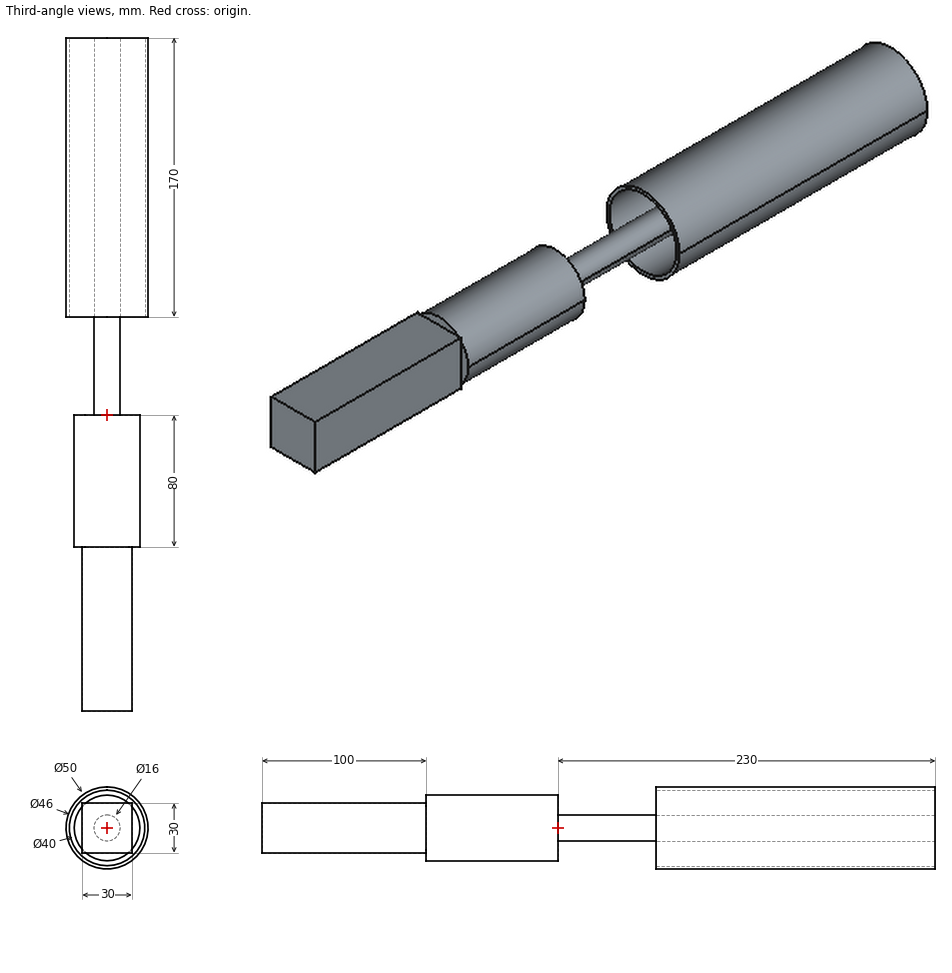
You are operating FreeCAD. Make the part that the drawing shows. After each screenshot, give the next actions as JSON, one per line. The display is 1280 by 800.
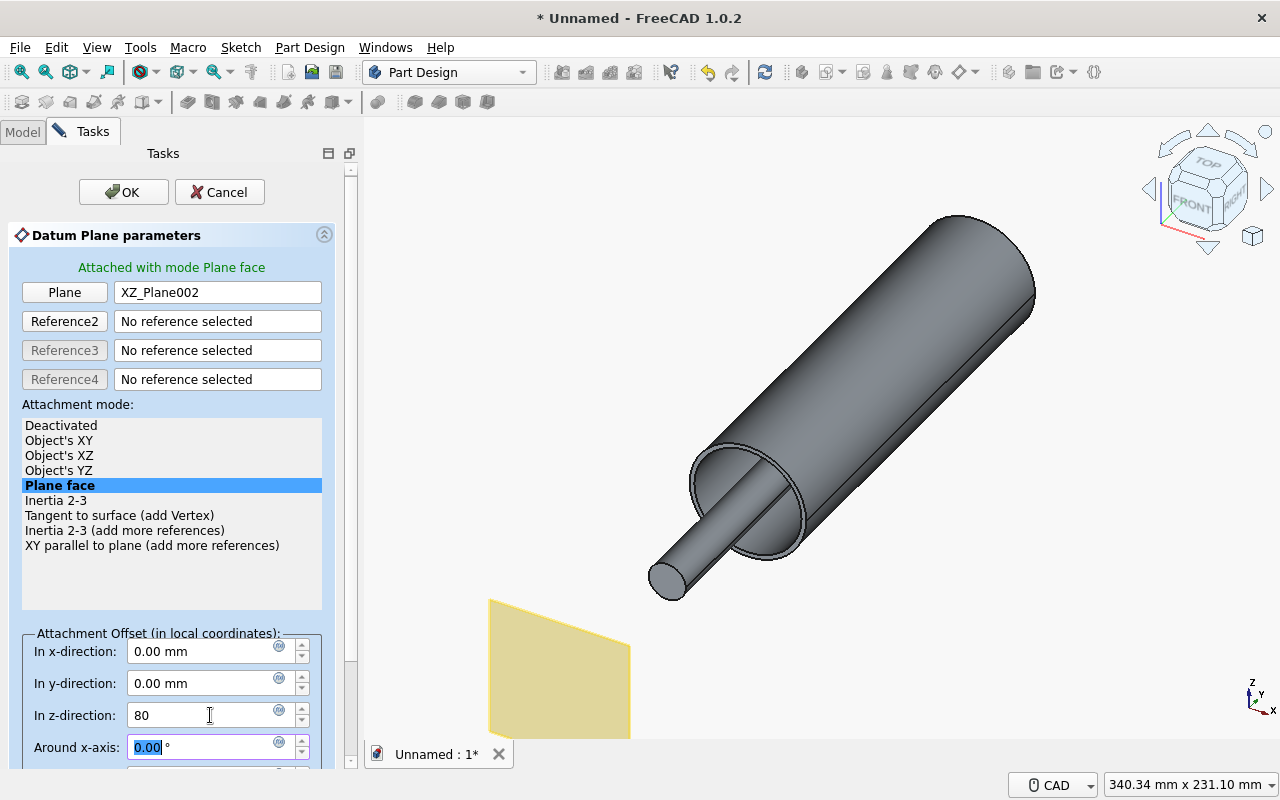
{"action": "left_click", "coordinate": [124, 192]}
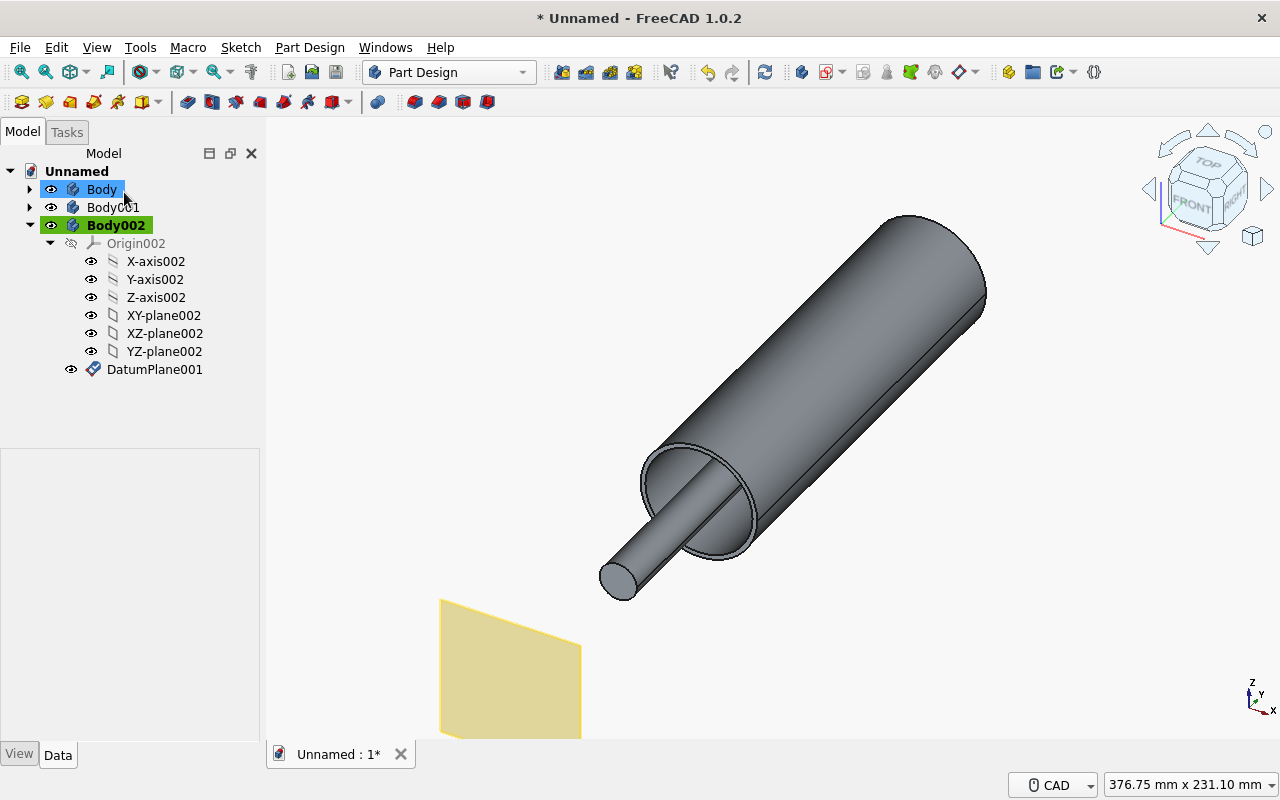
{"action": "left_click", "coordinate": [116, 369]}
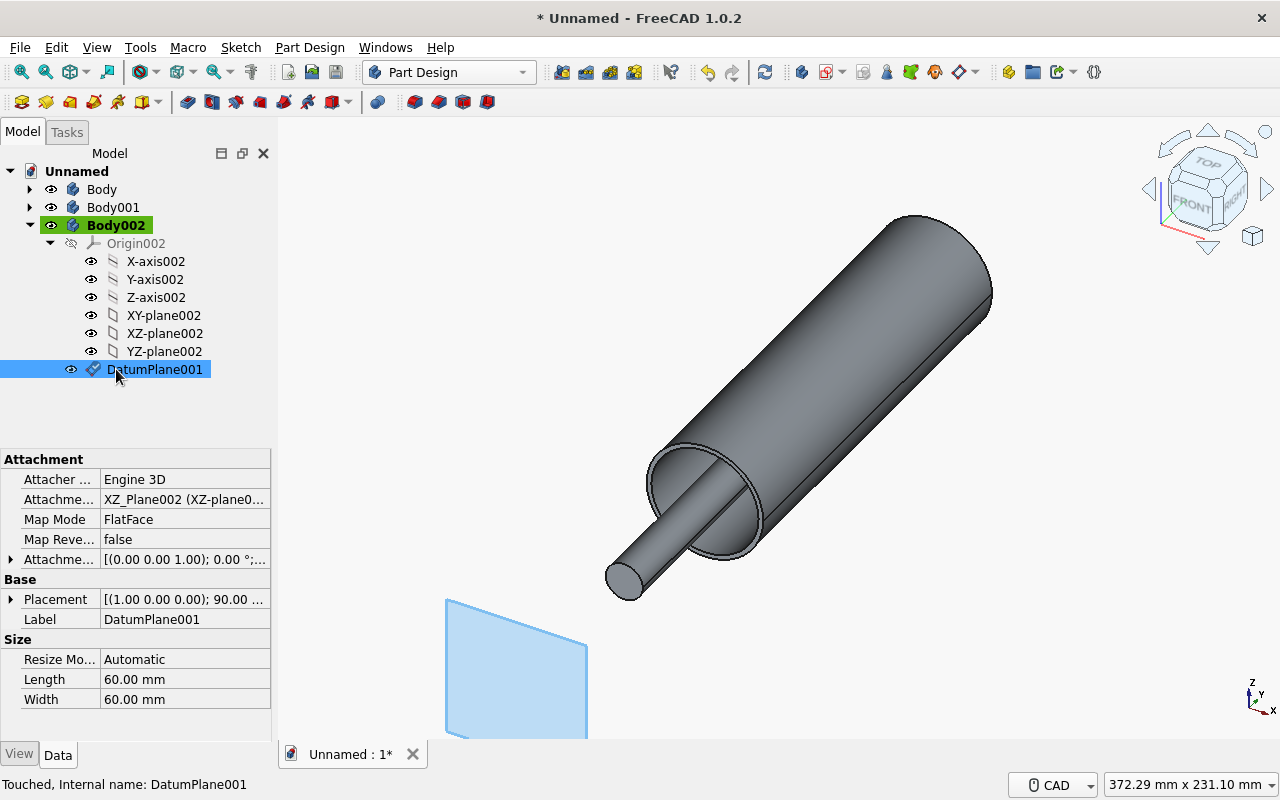
{"action": "left_click", "coordinate": [826, 72]}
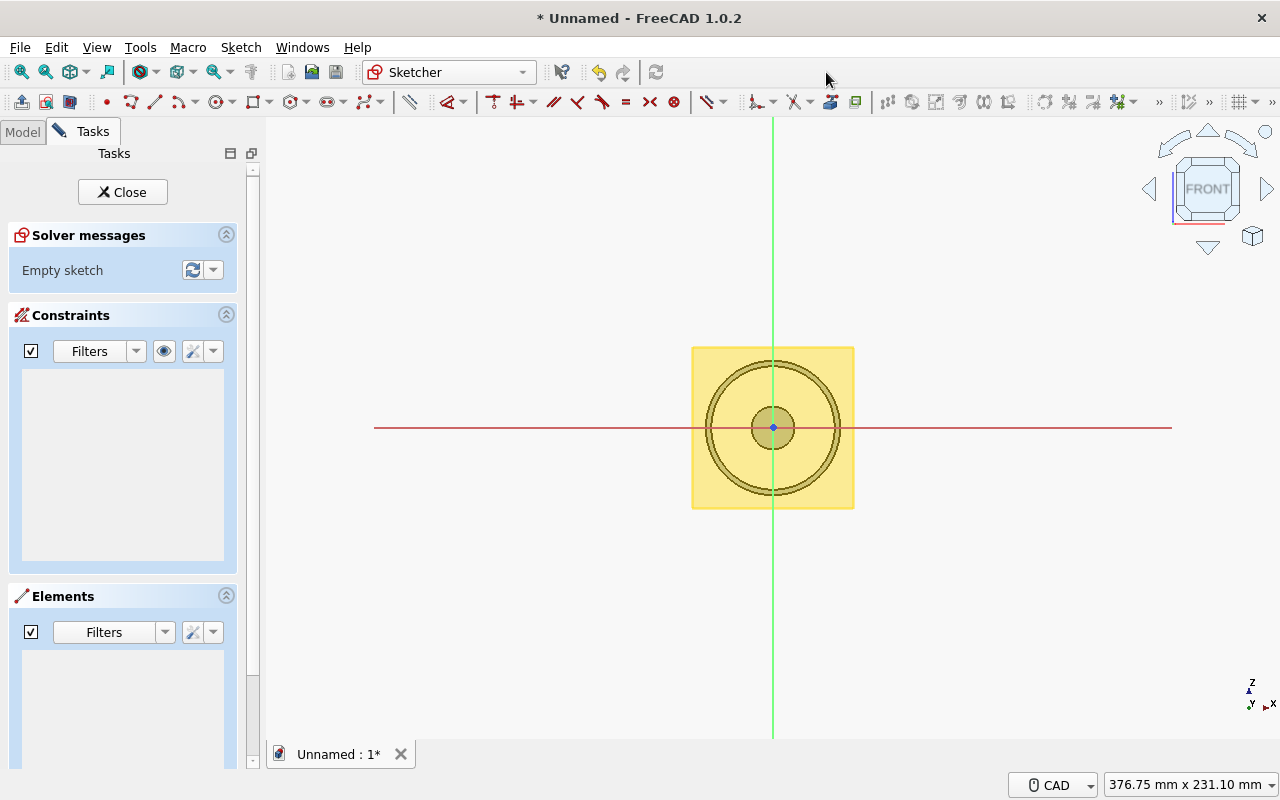
{"action": "scroll", "coordinate": [790, 428], "scroll_direction": "up", "scroll_amount": 8}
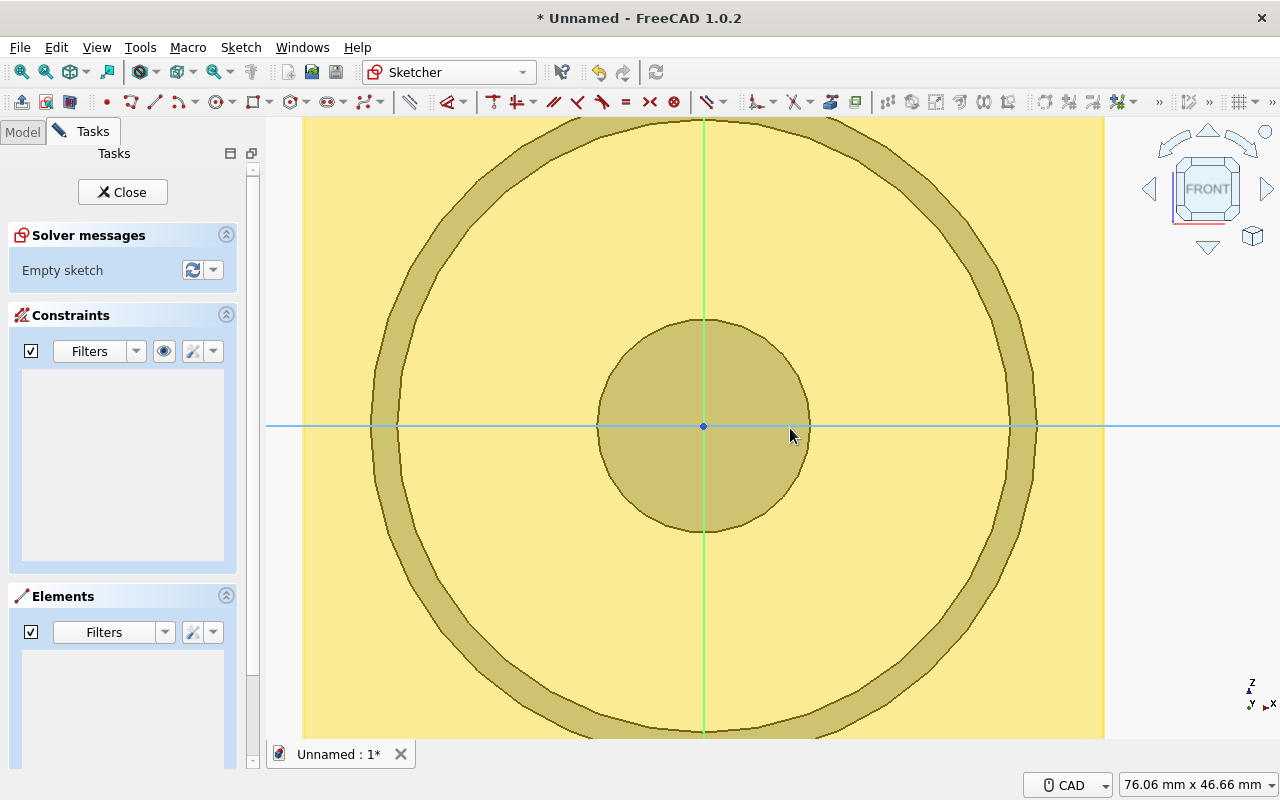
{"action": "key", "text": "g v"}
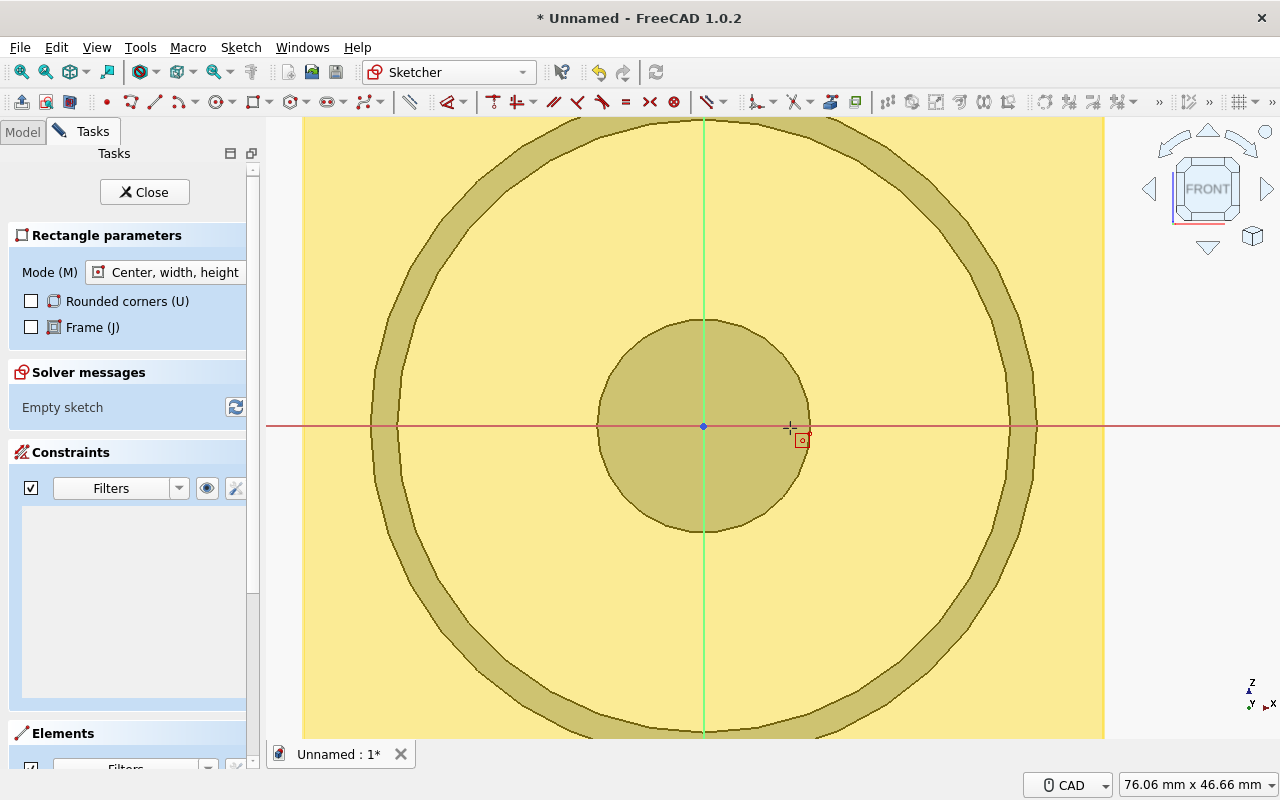
{"action": "left_click", "coordinate": [704, 426]}
{"action": "mouse_move", "coordinate": [904, 226]}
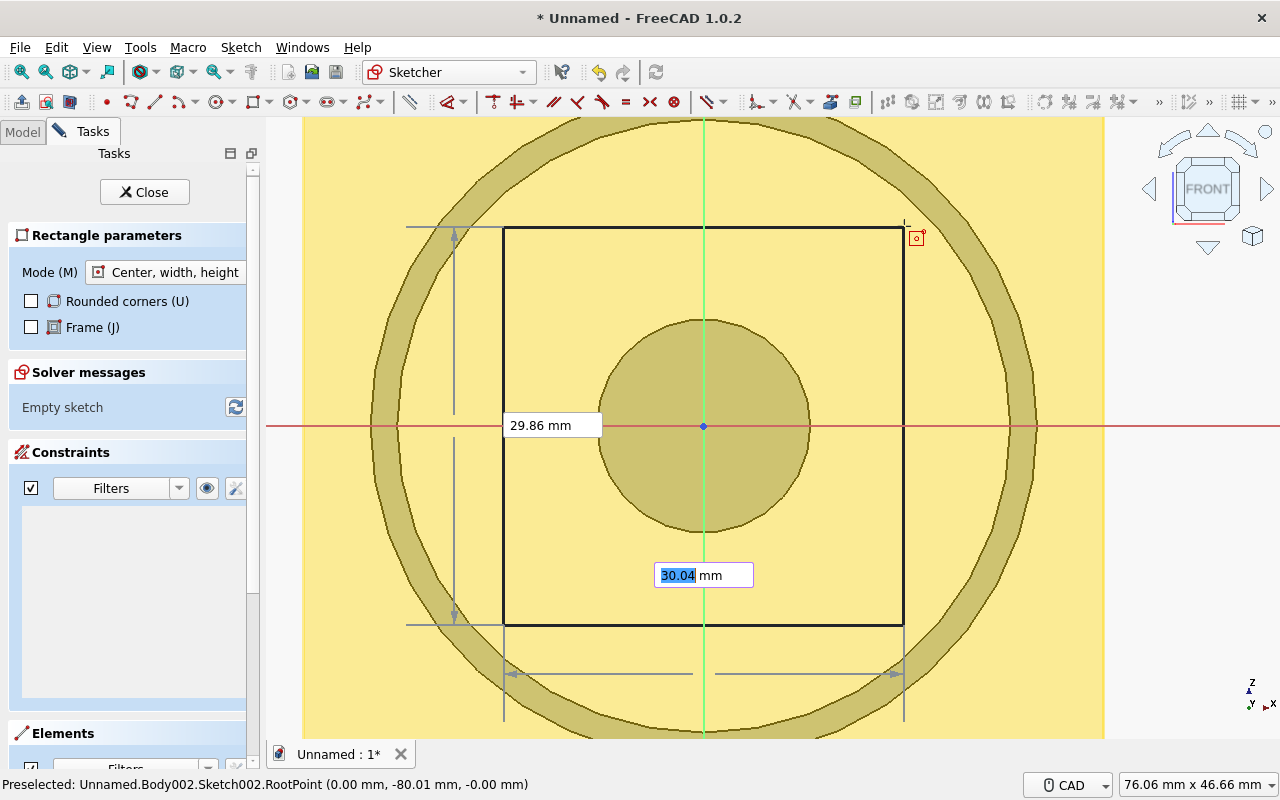
{"action": "type", "text": "30"}
{"action": "key", "text": "Tab"}
{"action": "type", "text": "30"}
{"action": "key", "text": "Return"}
{"action": "key", "text": "Escape"}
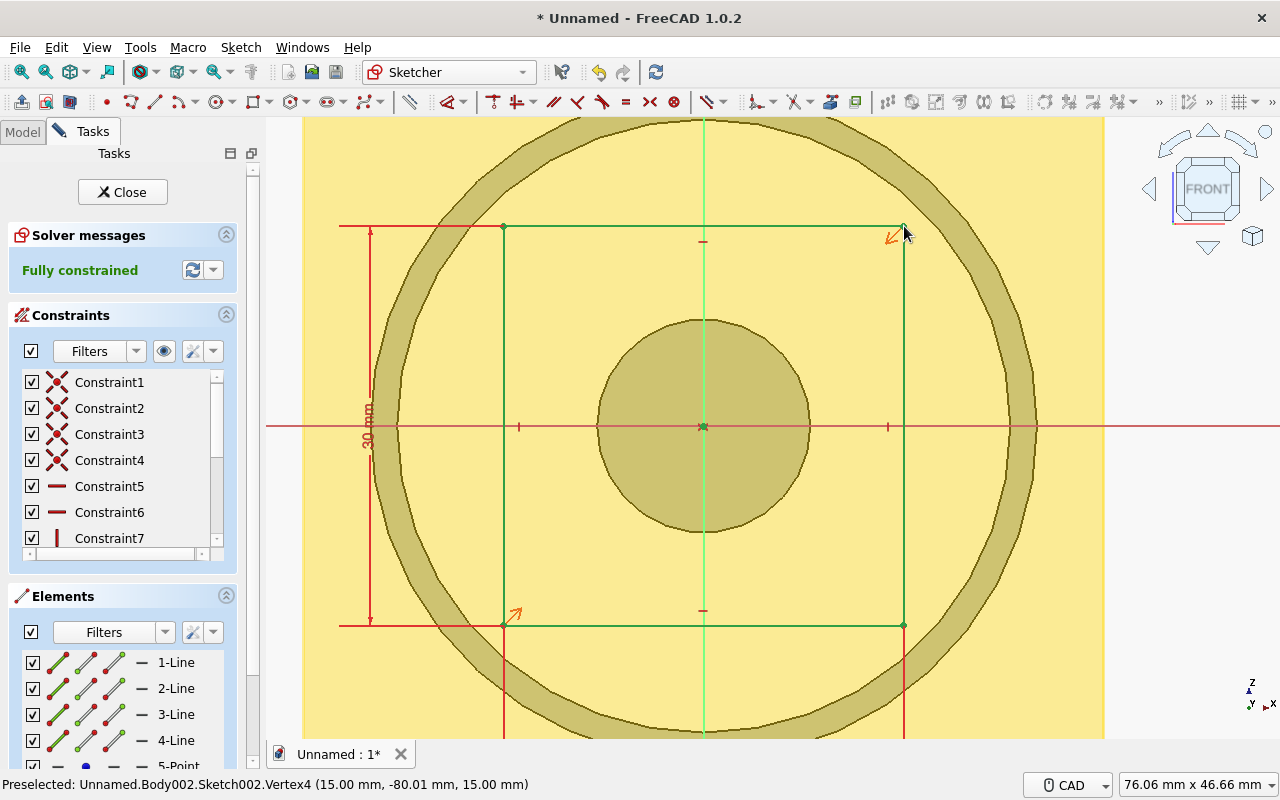
{"action": "left_click", "coordinate": [123, 192]}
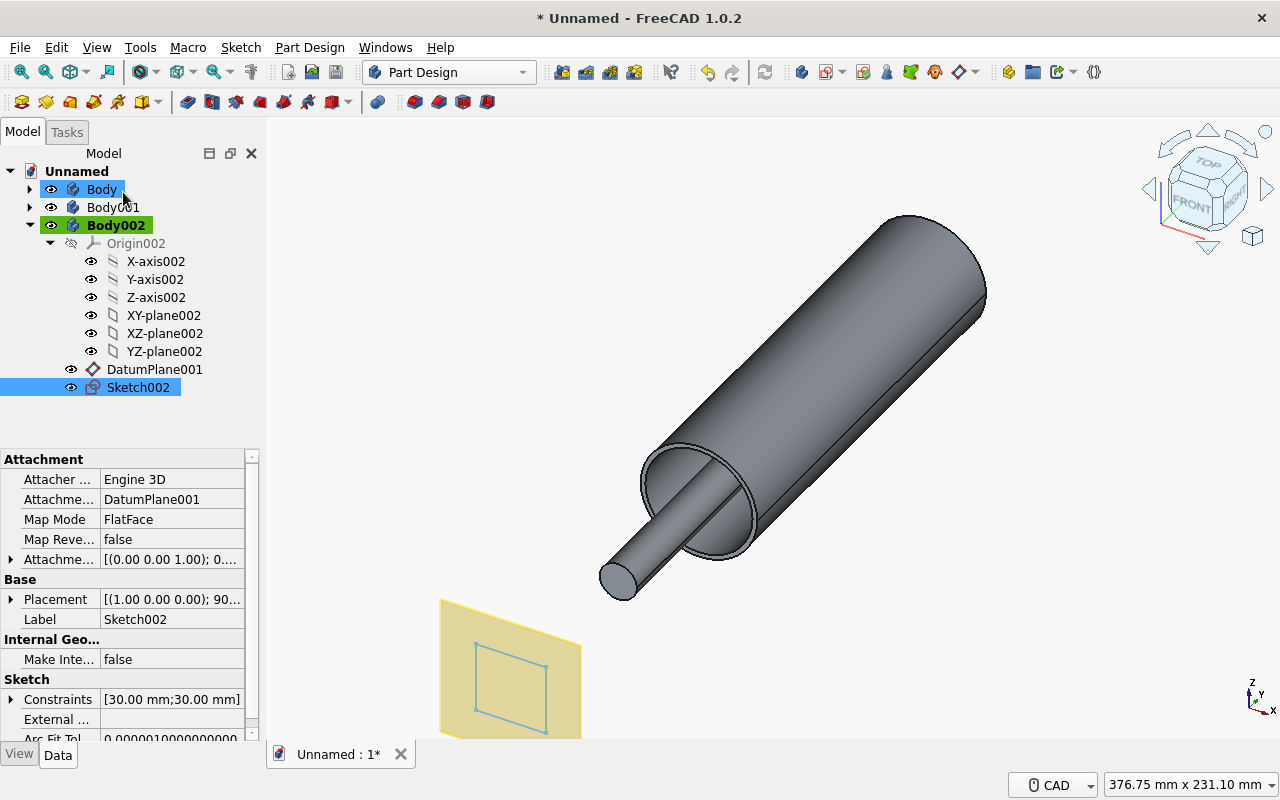
{"action": "left_click", "coordinate": [22, 102]}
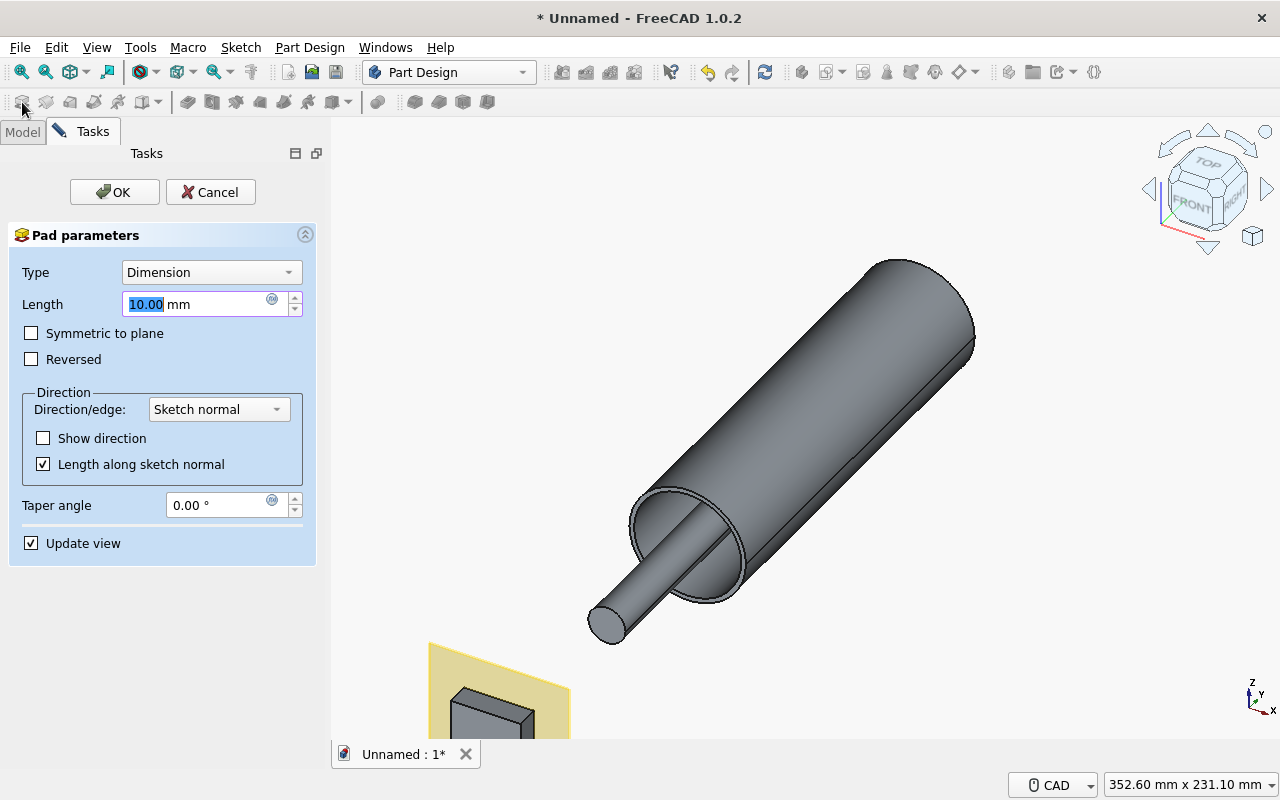
{"action": "type", "text": "100"}
{"action": "key", "text": "Tab"}